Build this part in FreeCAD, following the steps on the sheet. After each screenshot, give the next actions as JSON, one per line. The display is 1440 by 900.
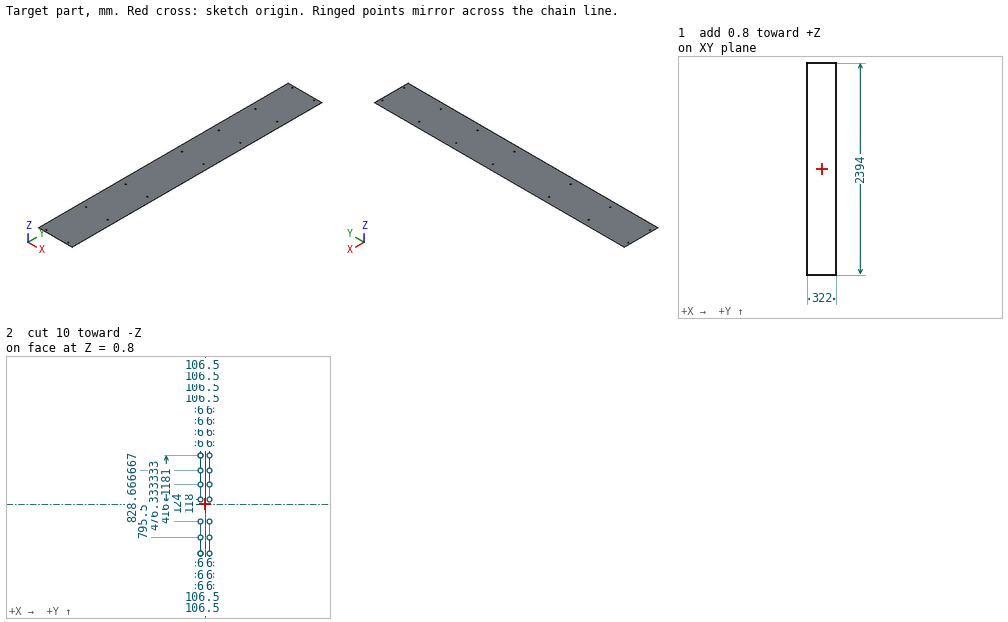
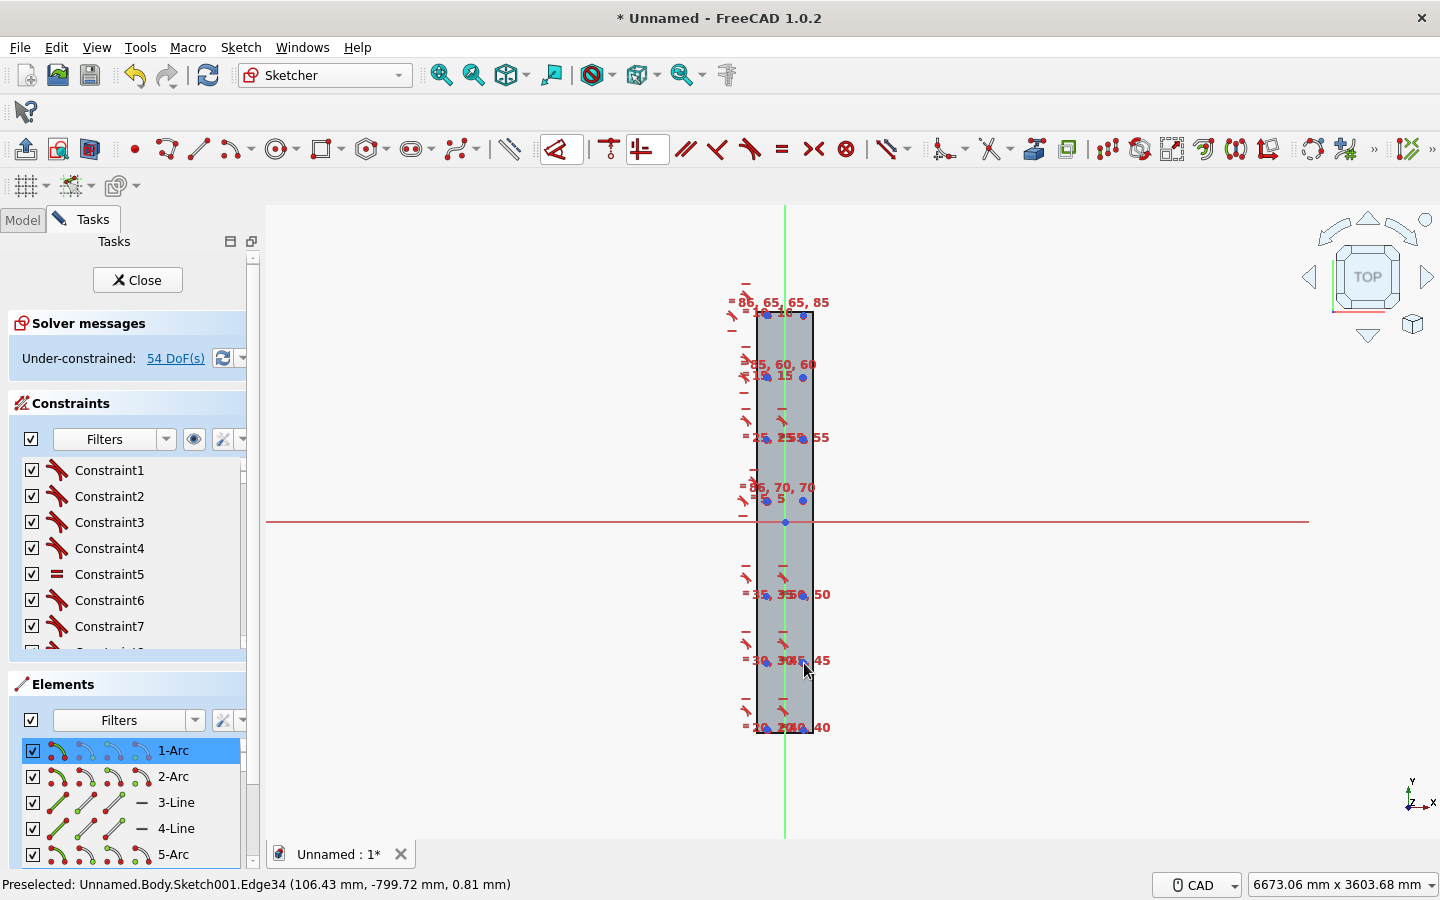
{"action": "scroll", "coordinate": [804, 596], "scroll_direction": "up", "scroll_amount": 14}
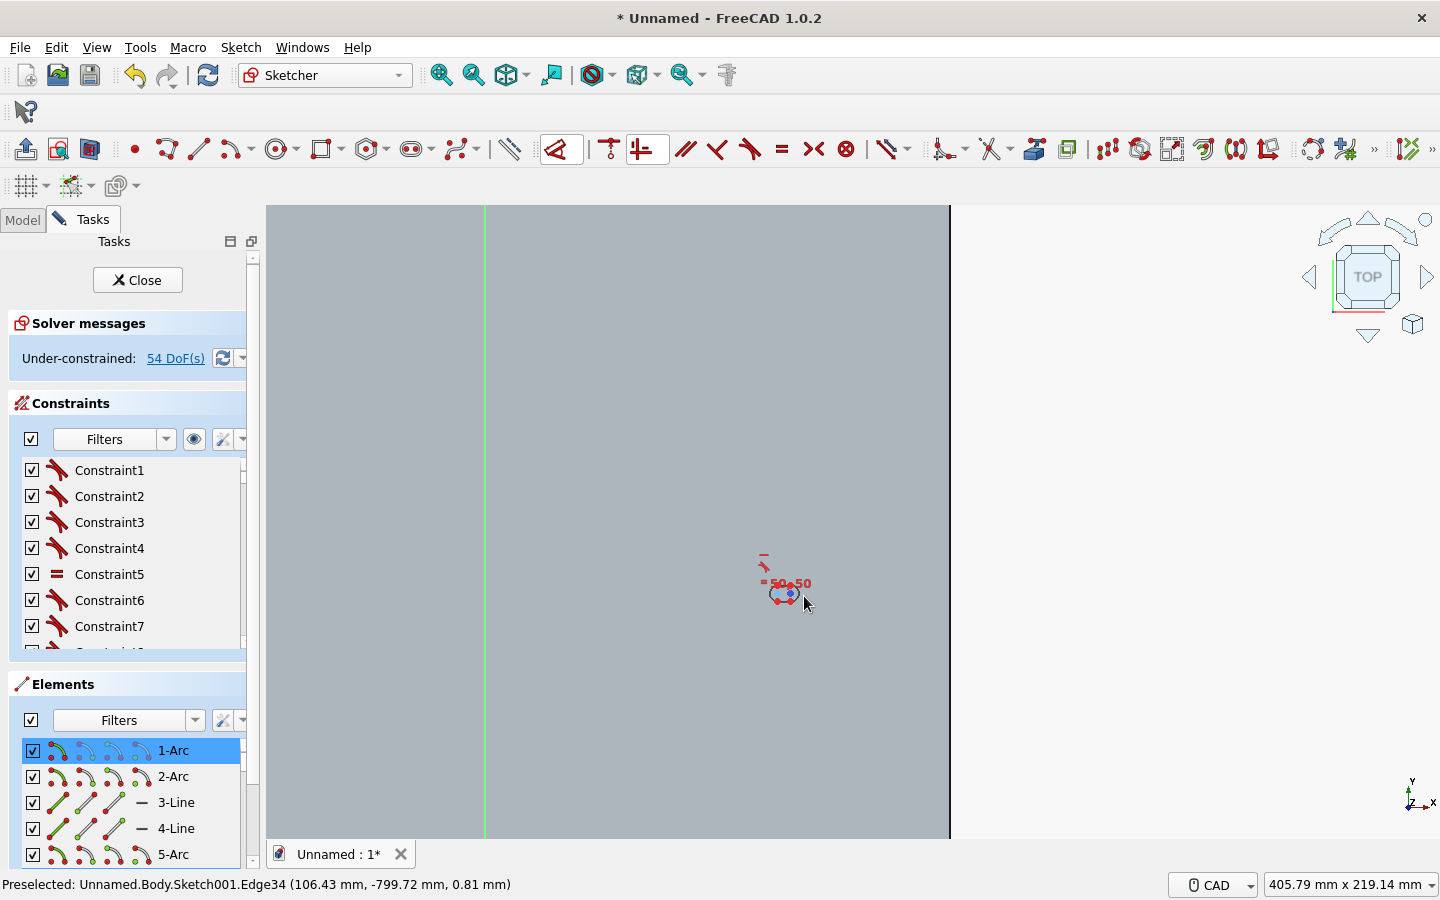
{"action": "left_click", "coordinate": [799, 594]}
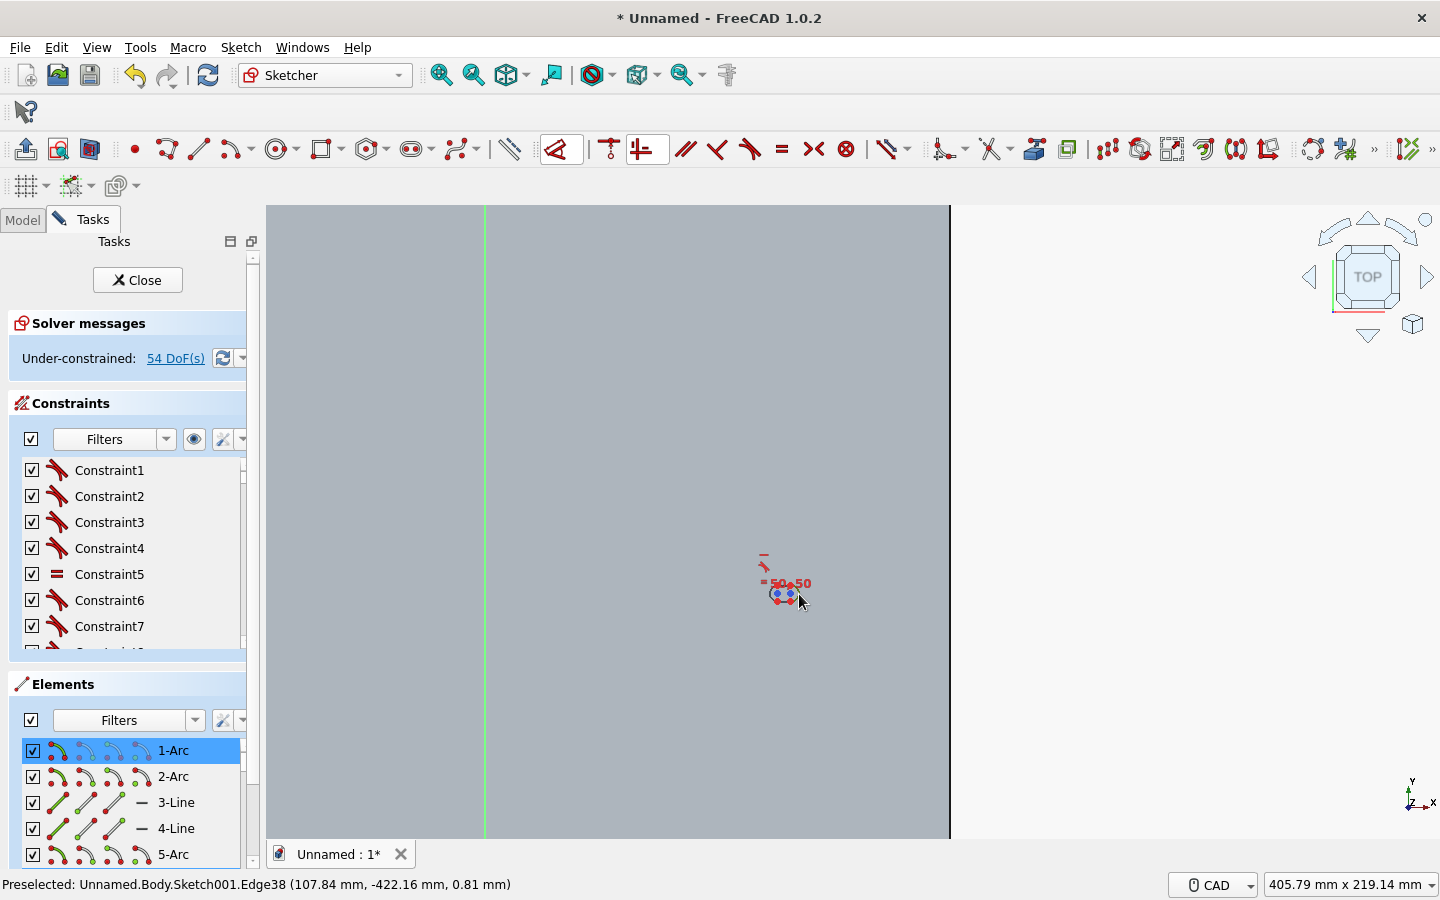
{"action": "scroll", "coordinate": [804, 596], "scroll_direction": "down", "scroll_amount": 14}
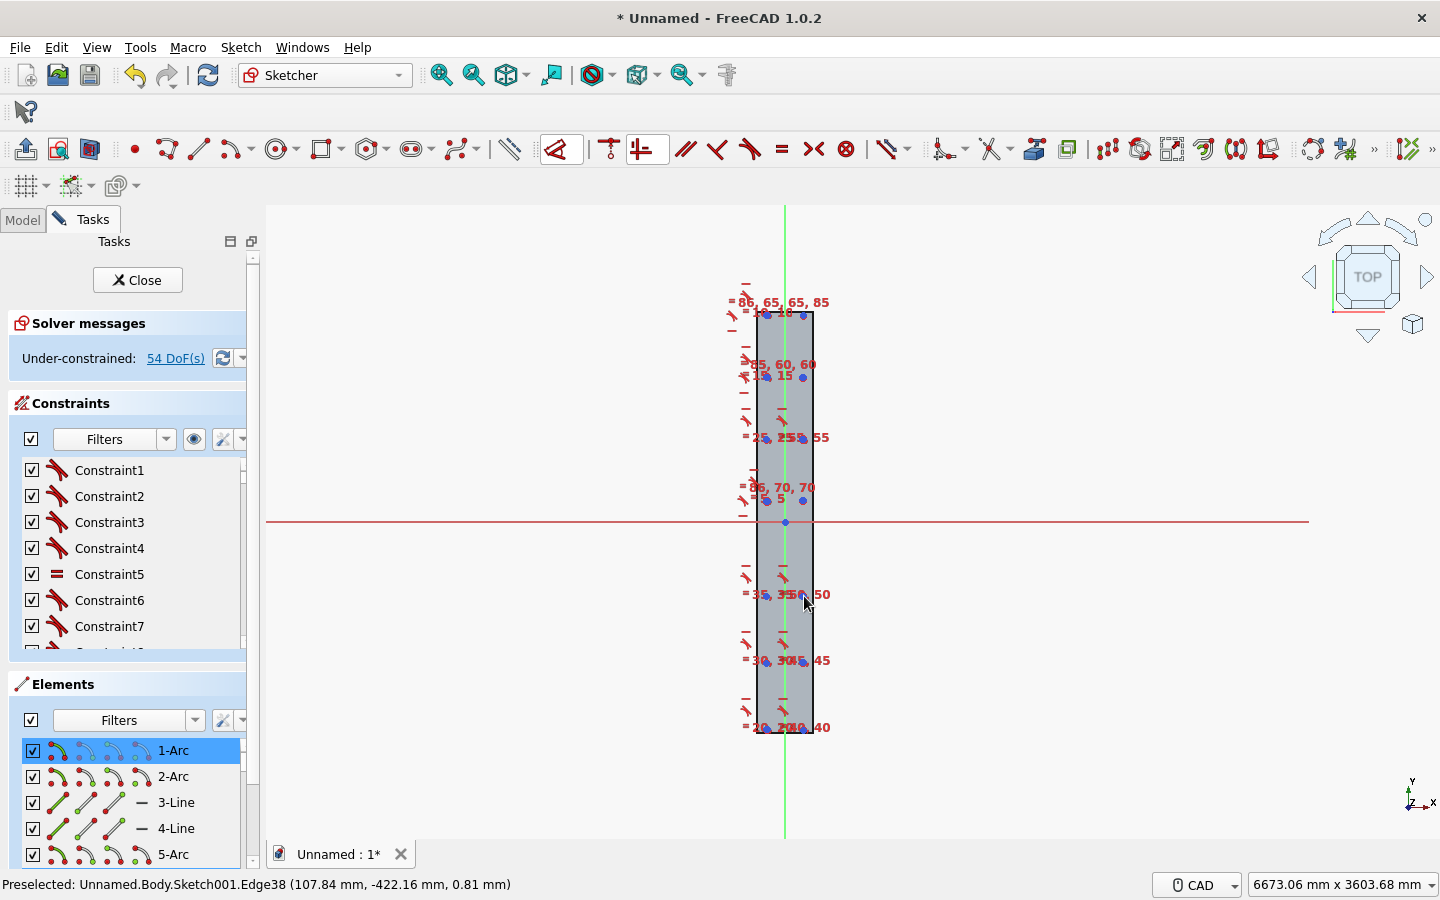
{"action": "scroll", "coordinate": [804, 440], "scroll_direction": "up", "scroll_amount": 14}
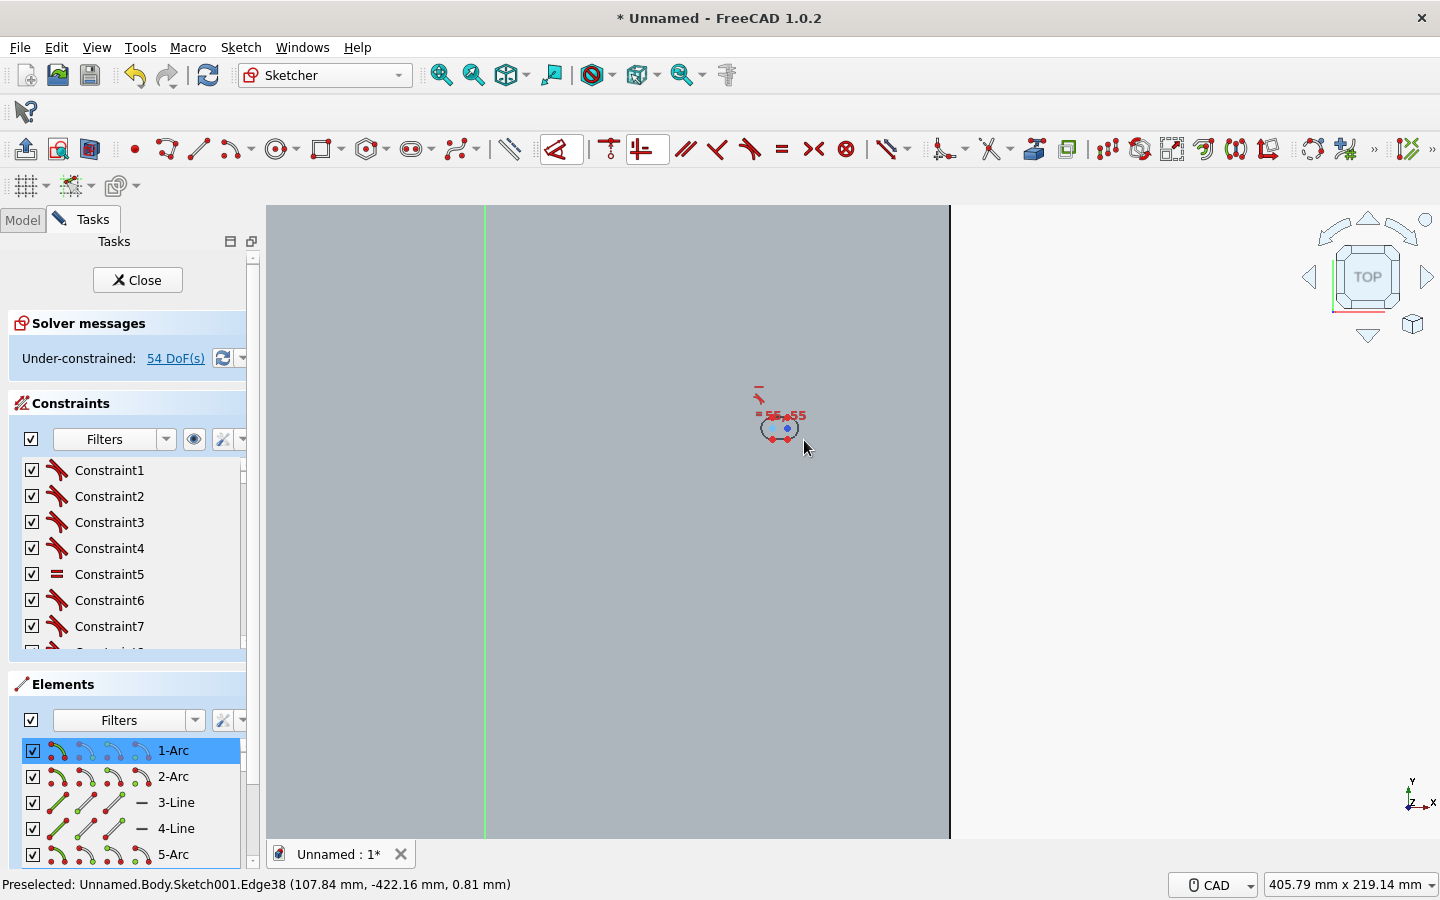
{"action": "left_click", "coordinate": [796, 435]}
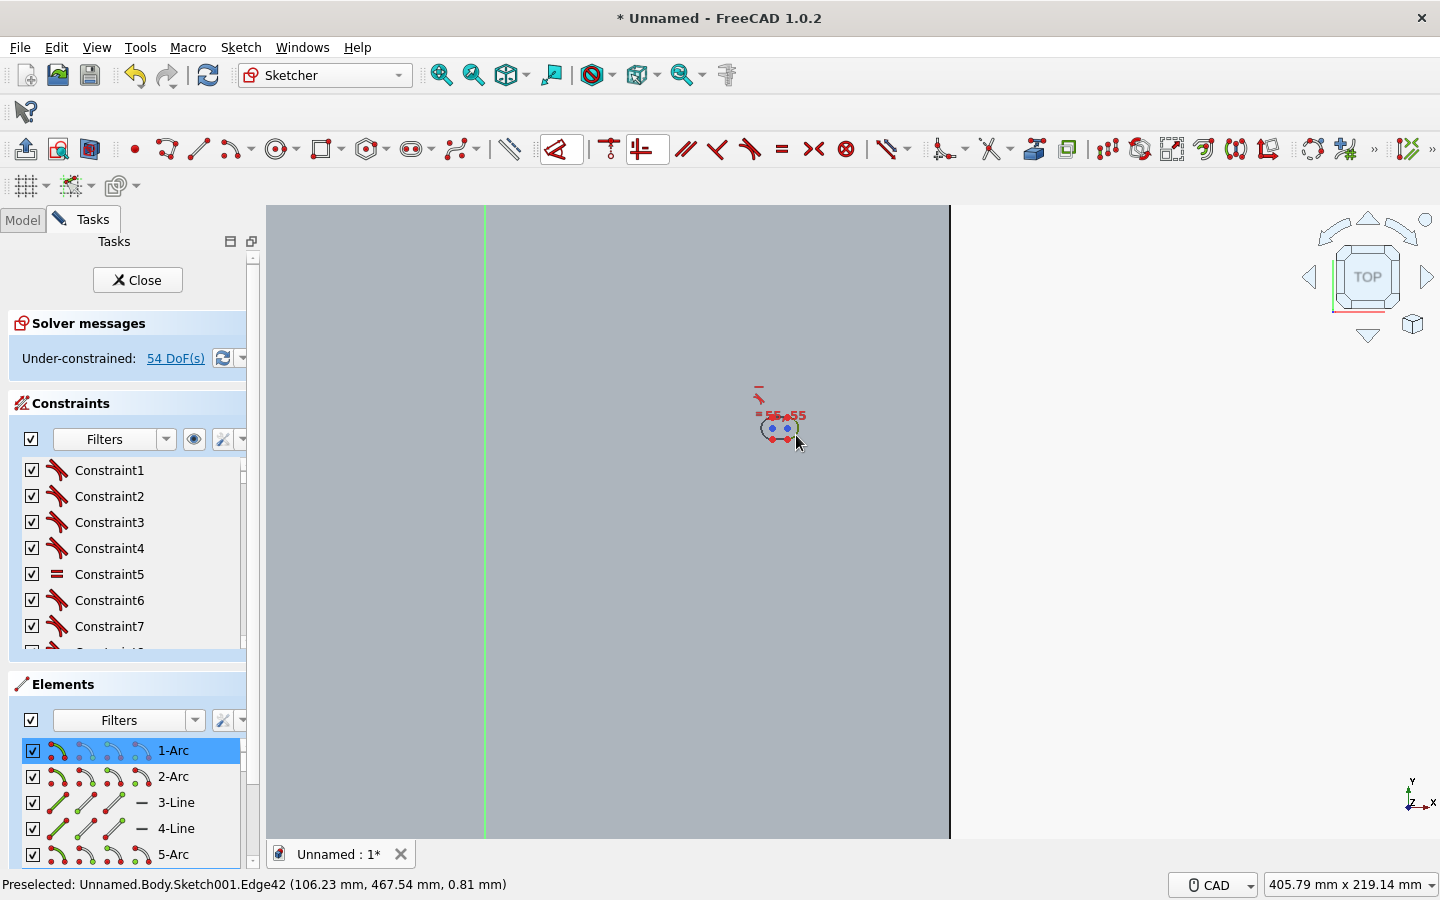
{"action": "scroll", "coordinate": [804, 440], "scroll_direction": "down", "scroll_amount": 14}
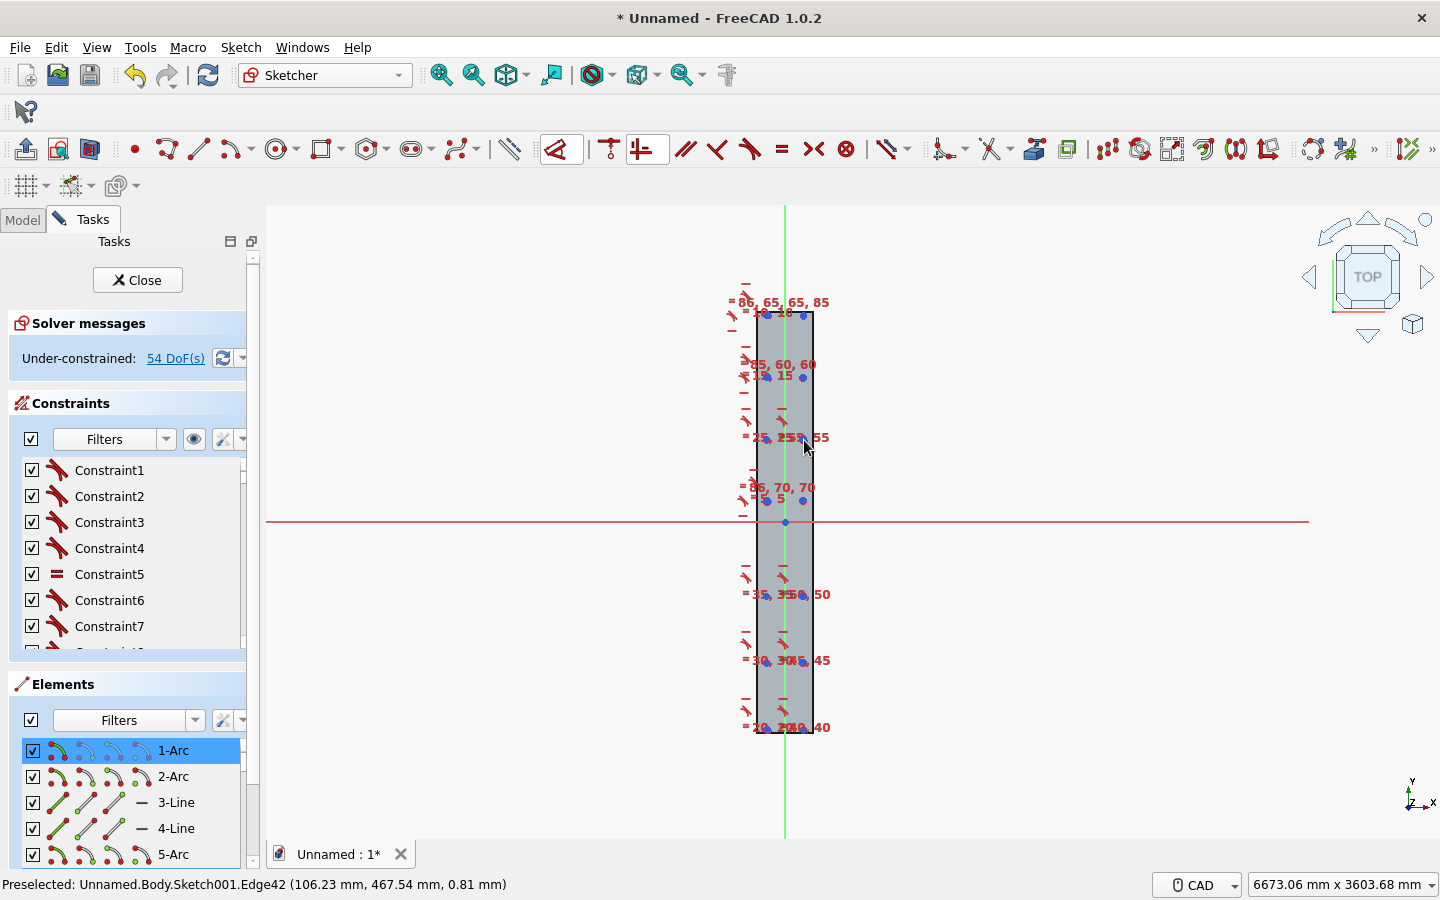
{"action": "scroll", "coordinate": [804, 378], "scroll_direction": "up", "scroll_amount": 14}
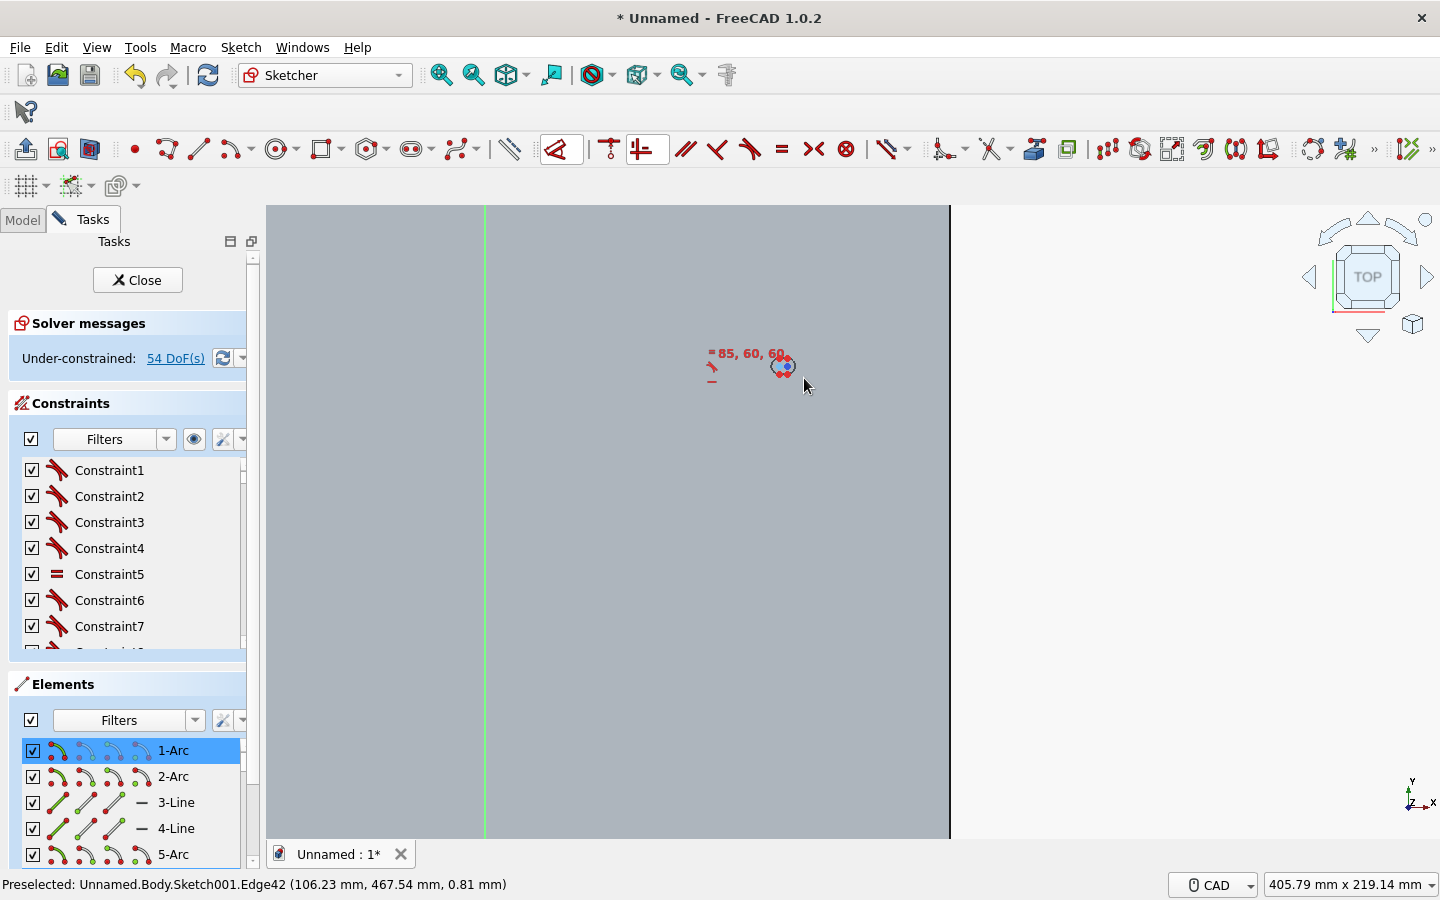
{"action": "left_click", "coordinate": [795, 366]}